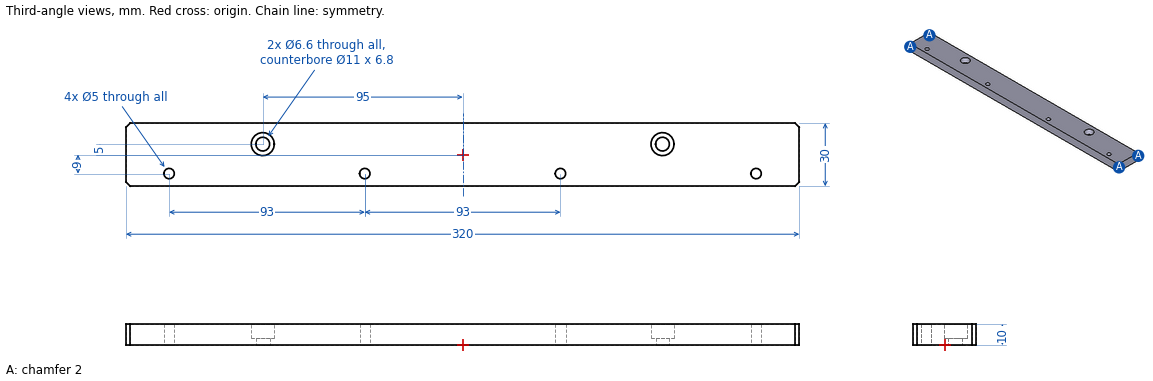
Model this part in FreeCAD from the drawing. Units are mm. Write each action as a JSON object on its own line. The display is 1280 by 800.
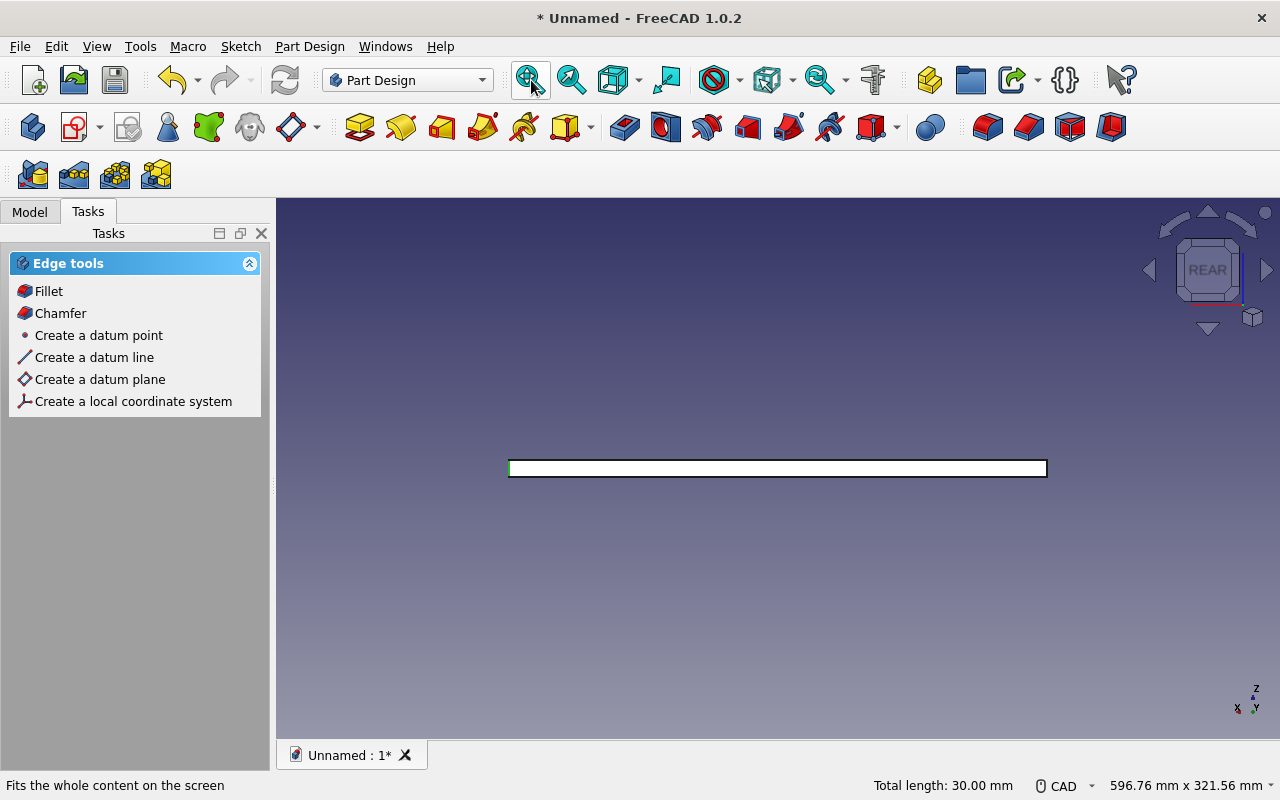
{"action": "left_click", "coordinate": [1047, 467], "text": "ctrl"}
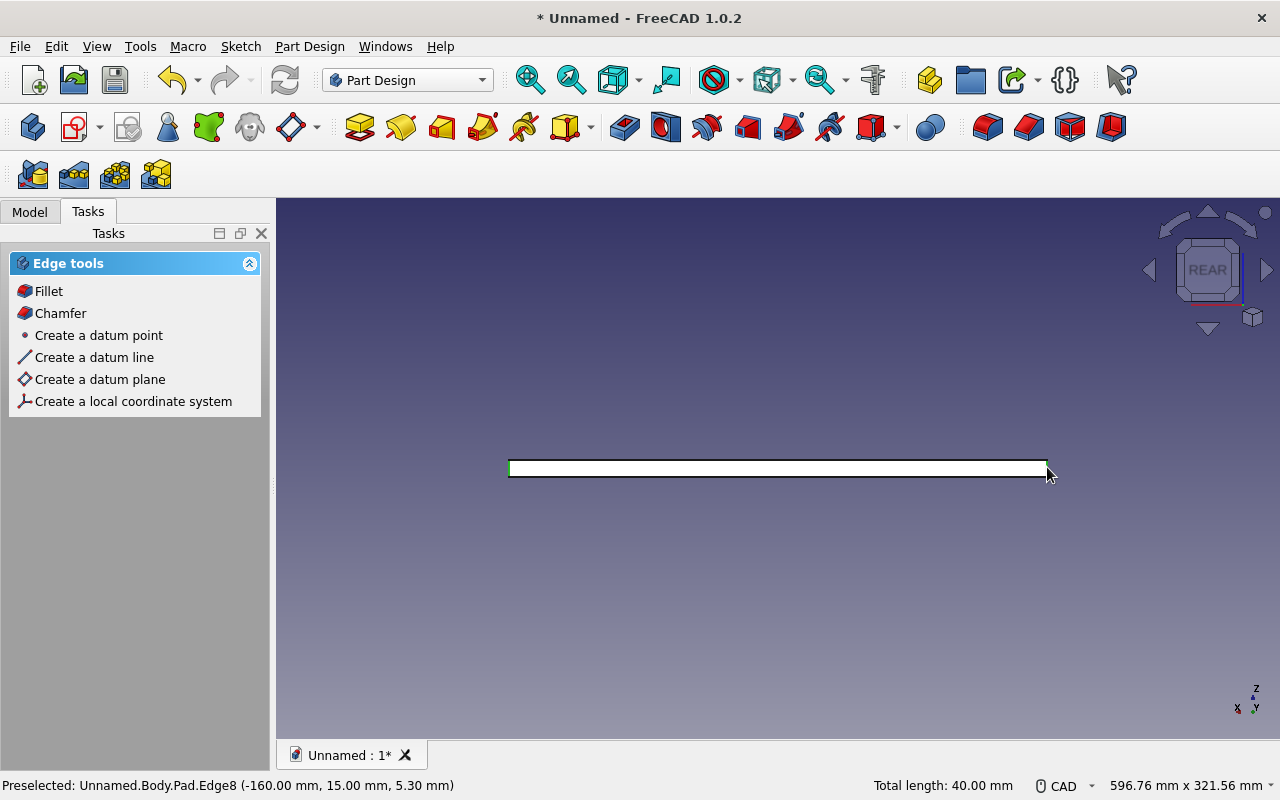
{"action": "left_click", "coordinate": [1029, 128]}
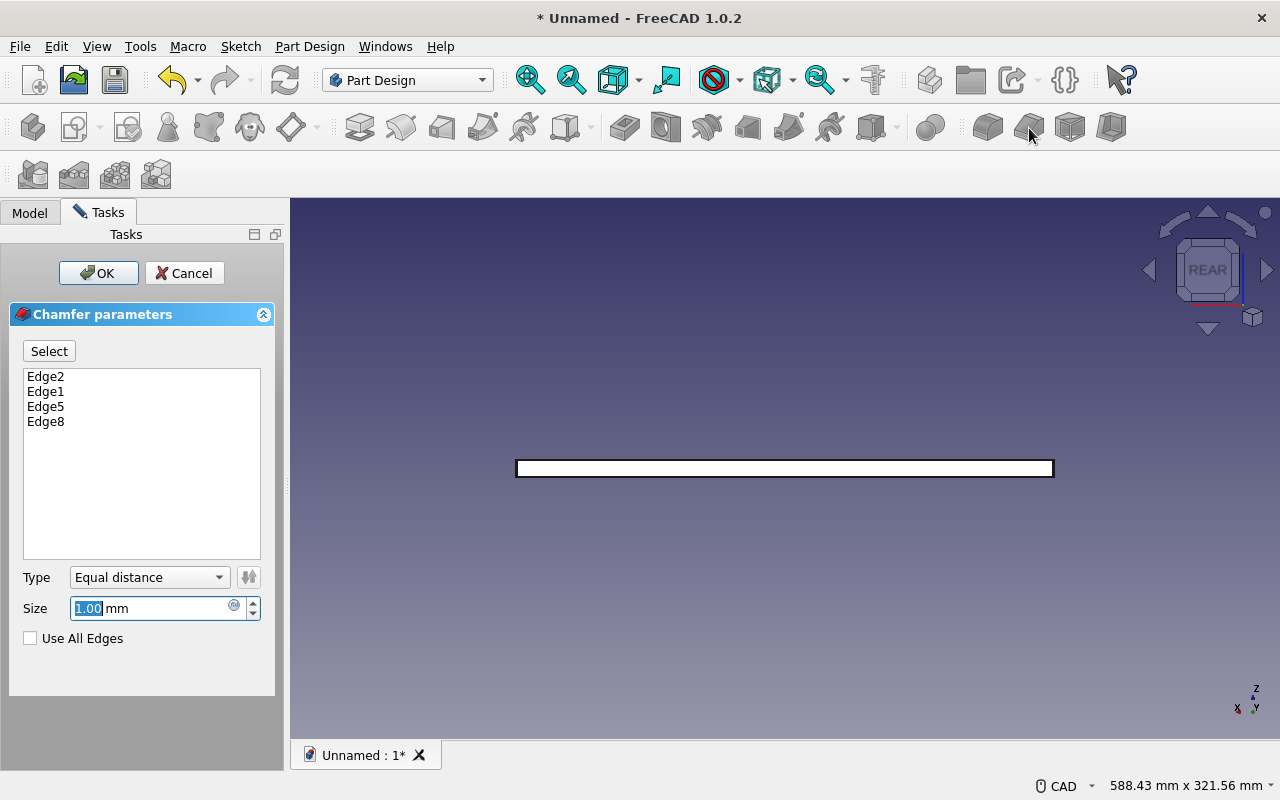
{"action": "type", "text": "2"}
{"action": "key", "text": "Tab"}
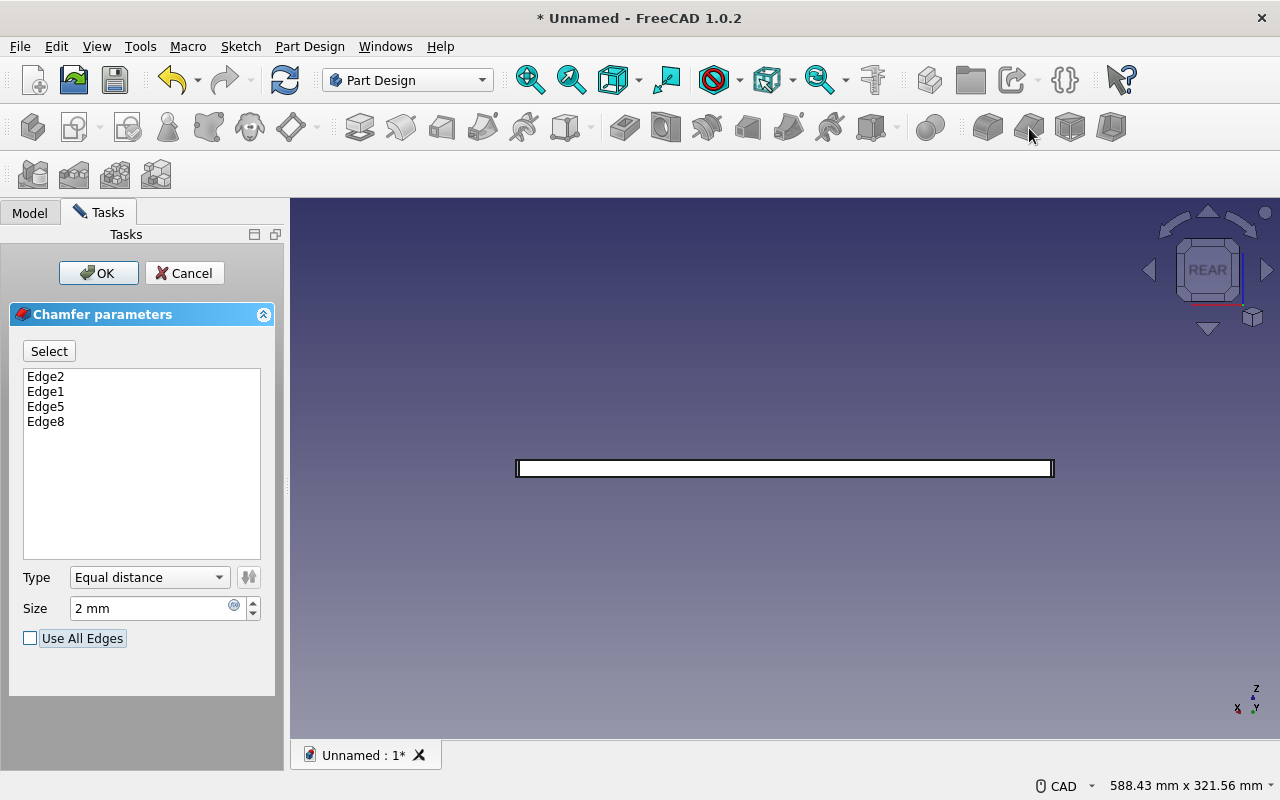
{"action": "left_click", "coordinate": [99, 273]}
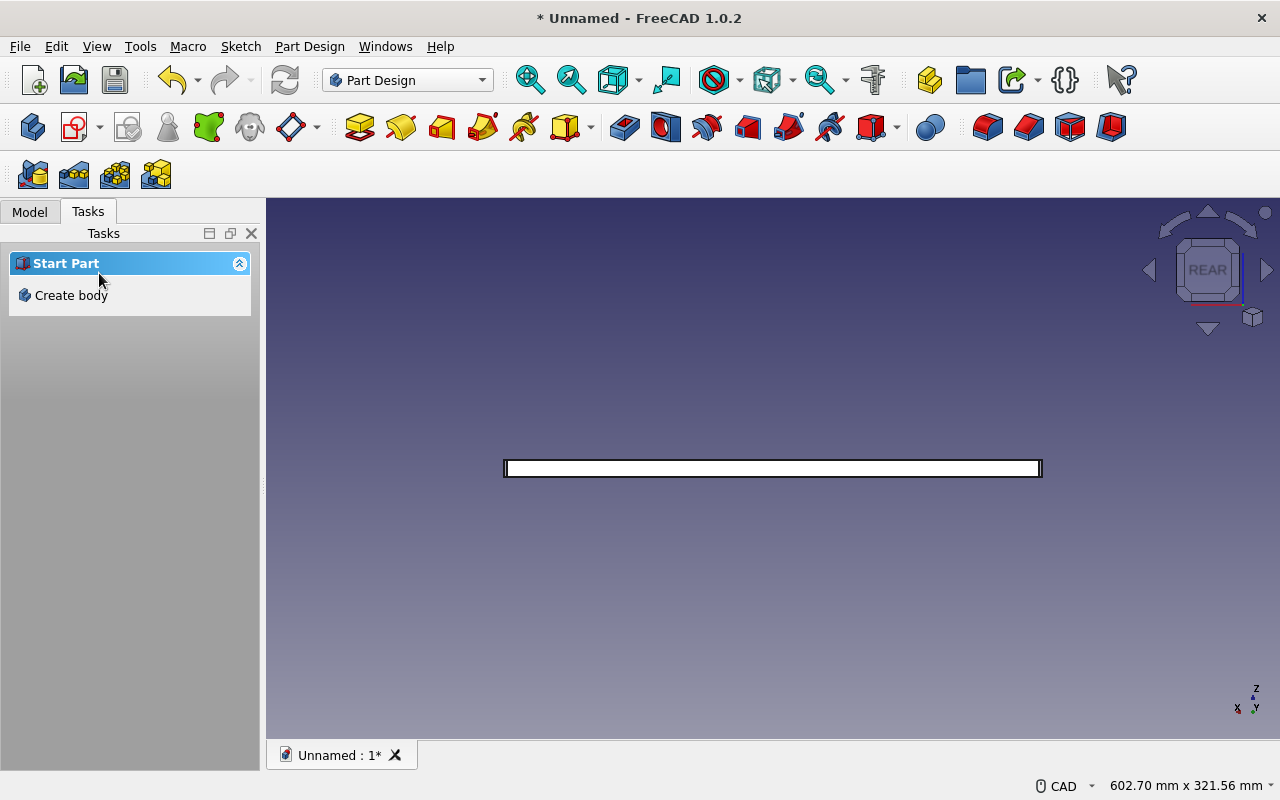
{"action": "key", "text": "0"}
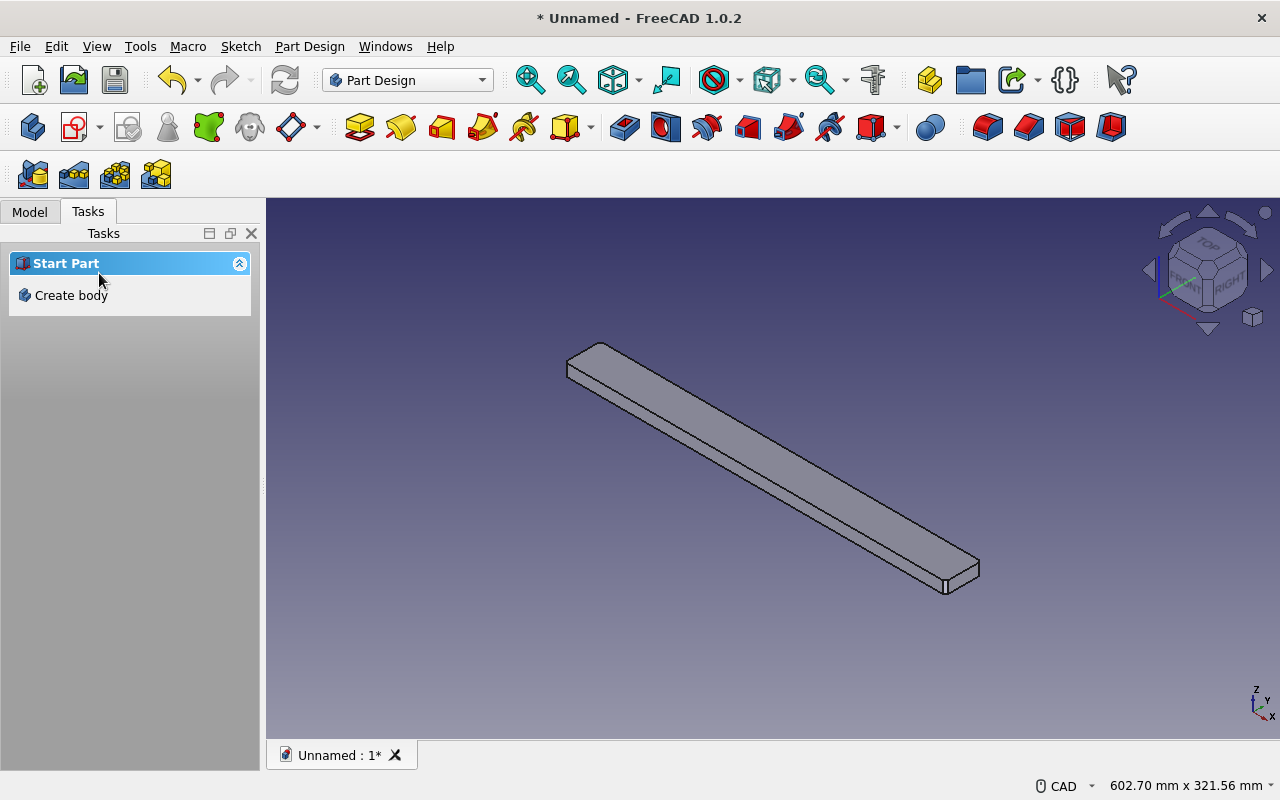
{"action": "left_click", "coordinate": [936, 555]}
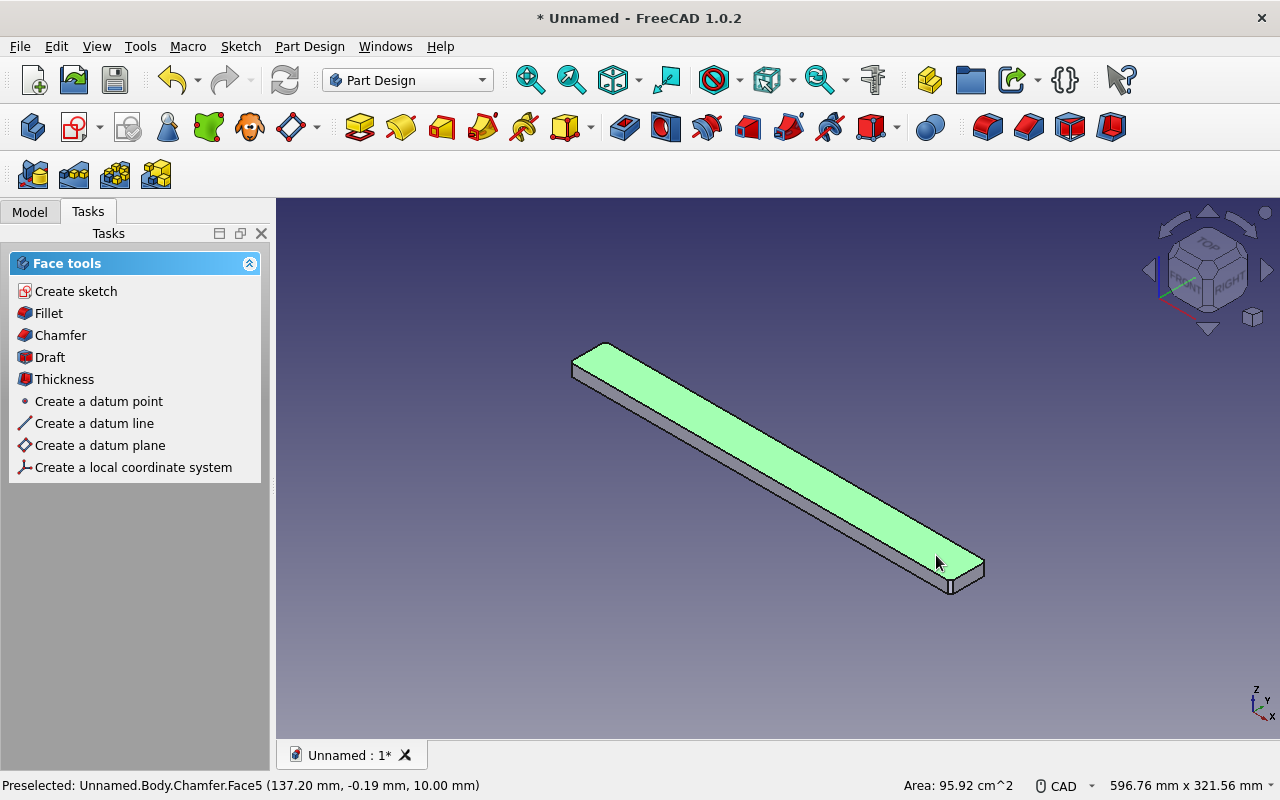
{"action": "left_click", "coordinate": [74, 128]}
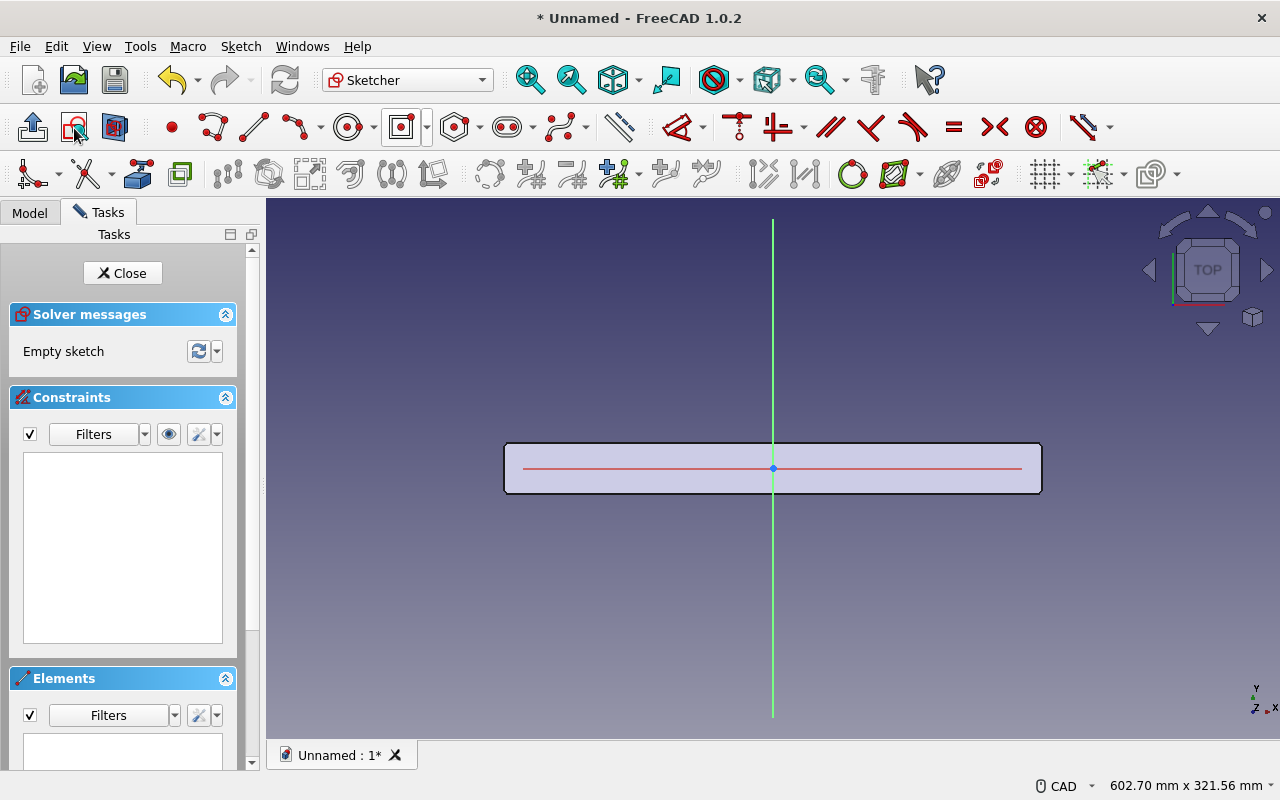
{"action": "left_click", "coordinate": [348, 128]}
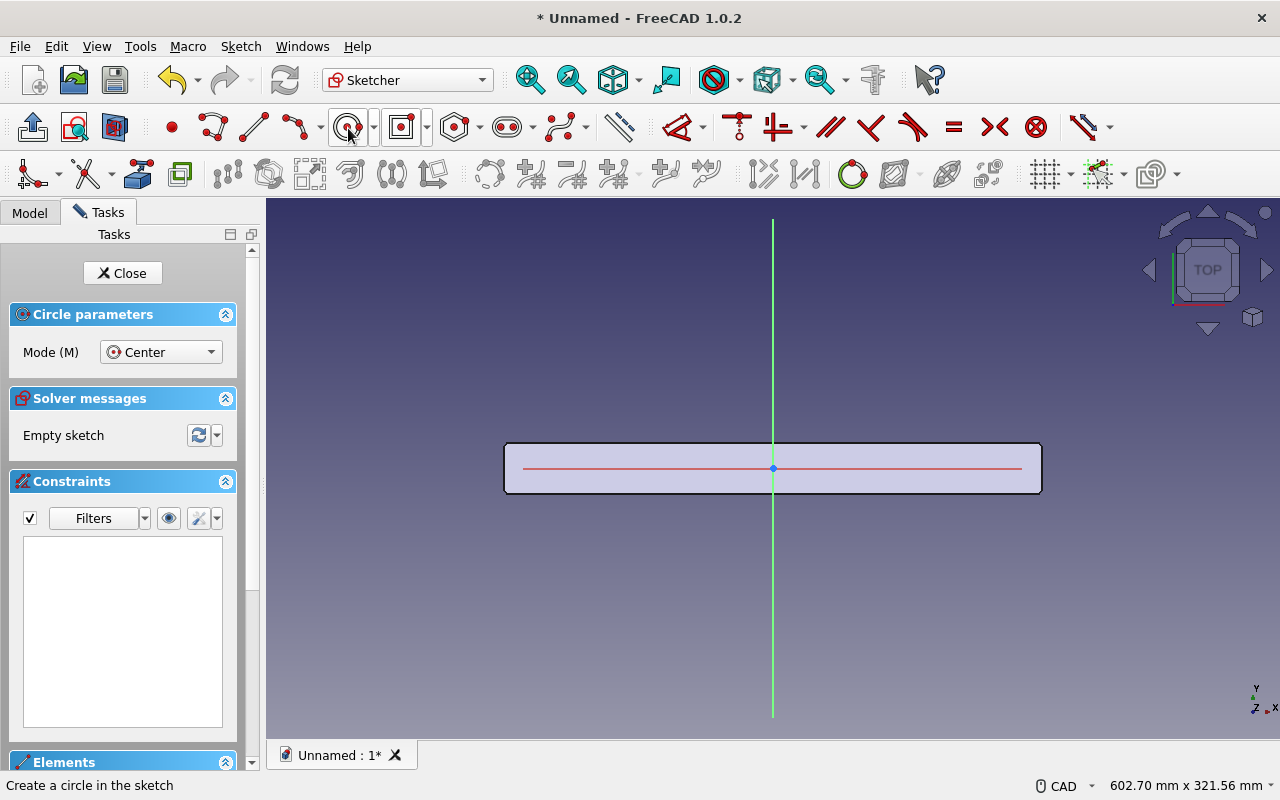
{"action": "scroll", "coordinate": [538, 484], "scroll_direction": "up", "scroll_amount": 9}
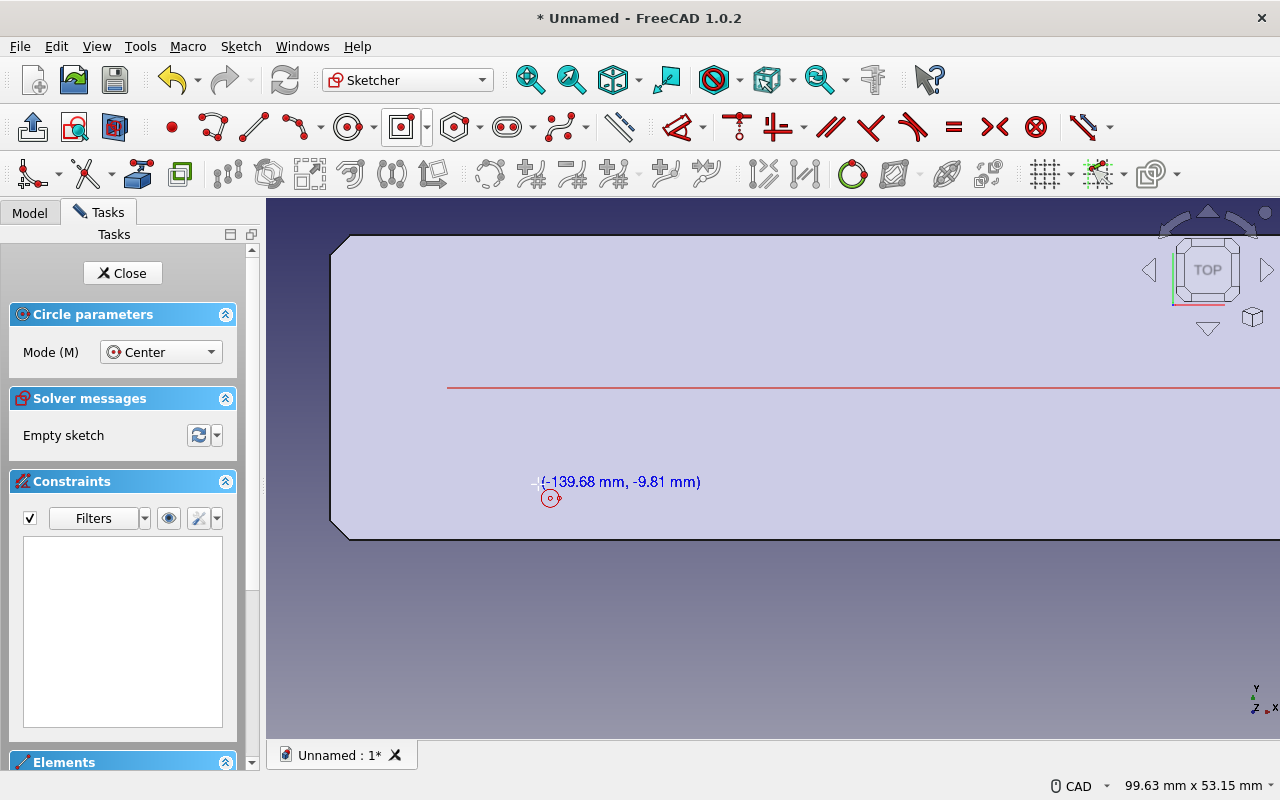
{"action": "scroll", "coordinate": [387, 474], "scroll_direction": "down", "scroll_amount": 8}